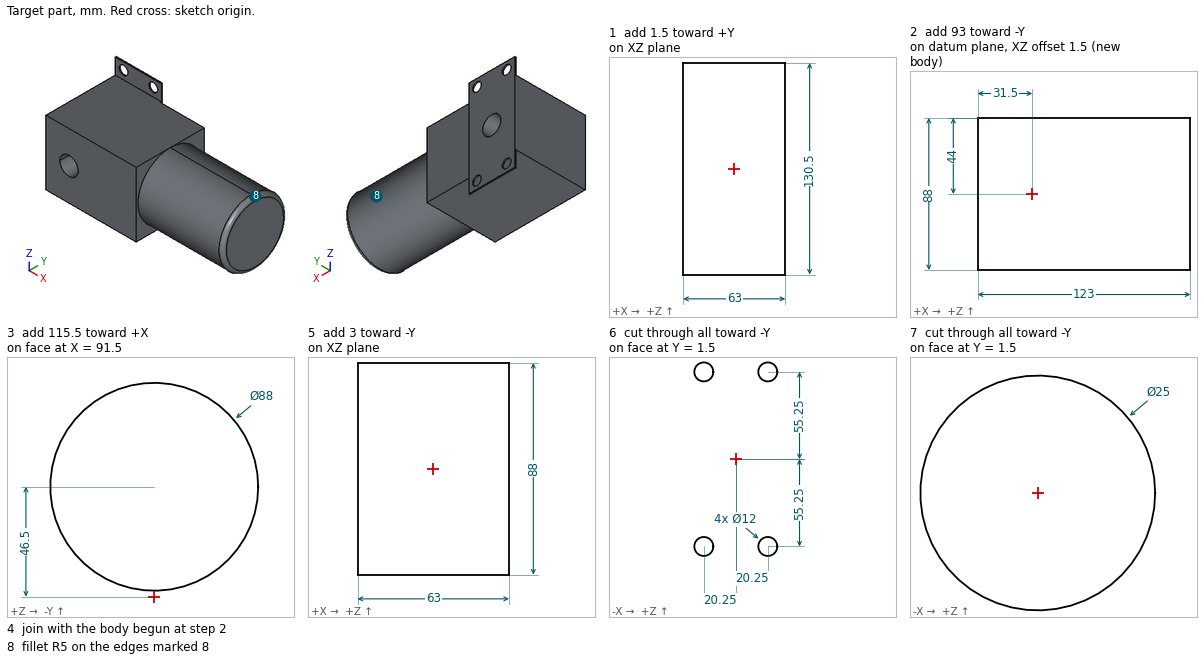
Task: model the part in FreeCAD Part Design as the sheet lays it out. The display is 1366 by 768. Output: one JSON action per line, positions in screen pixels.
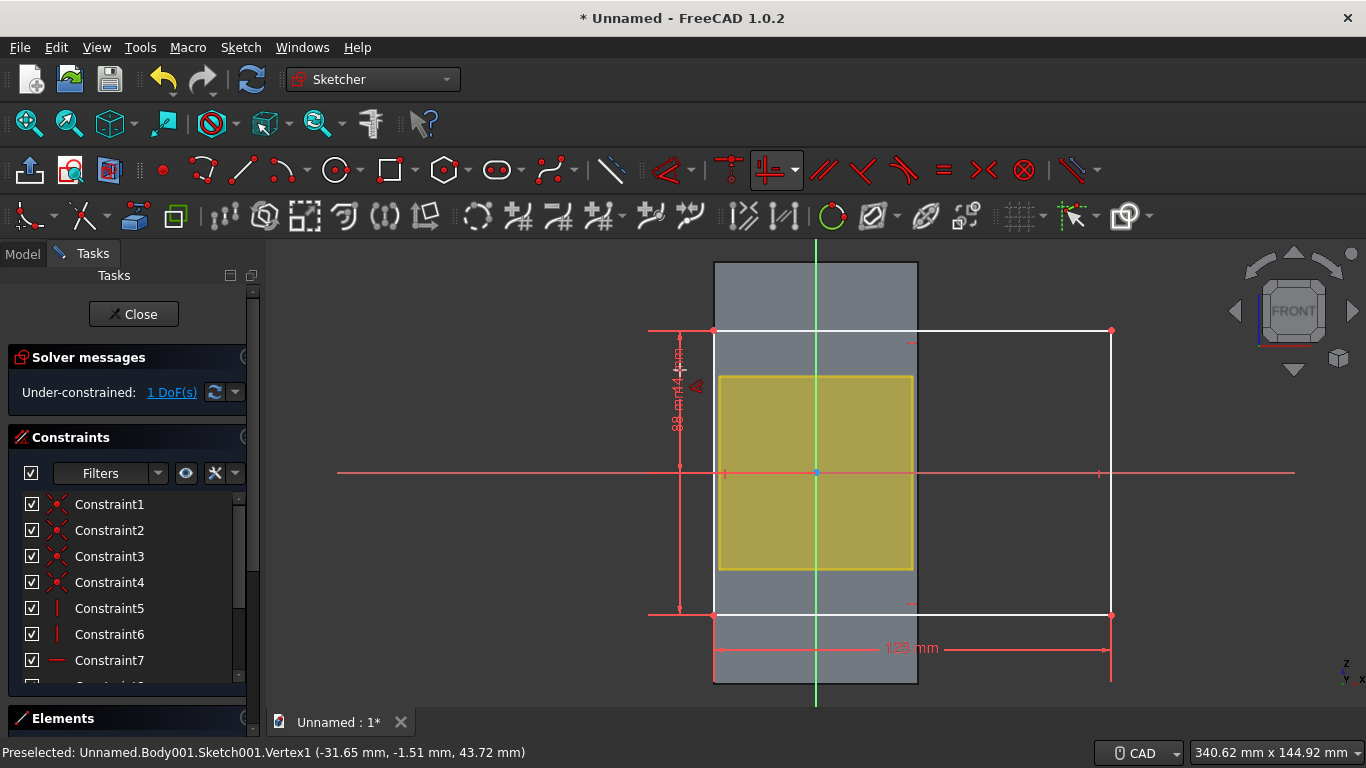
{"action": "left_click", "coordinate": [714, 331]}
{"action": "left_click", "coordinate": [765, 297]}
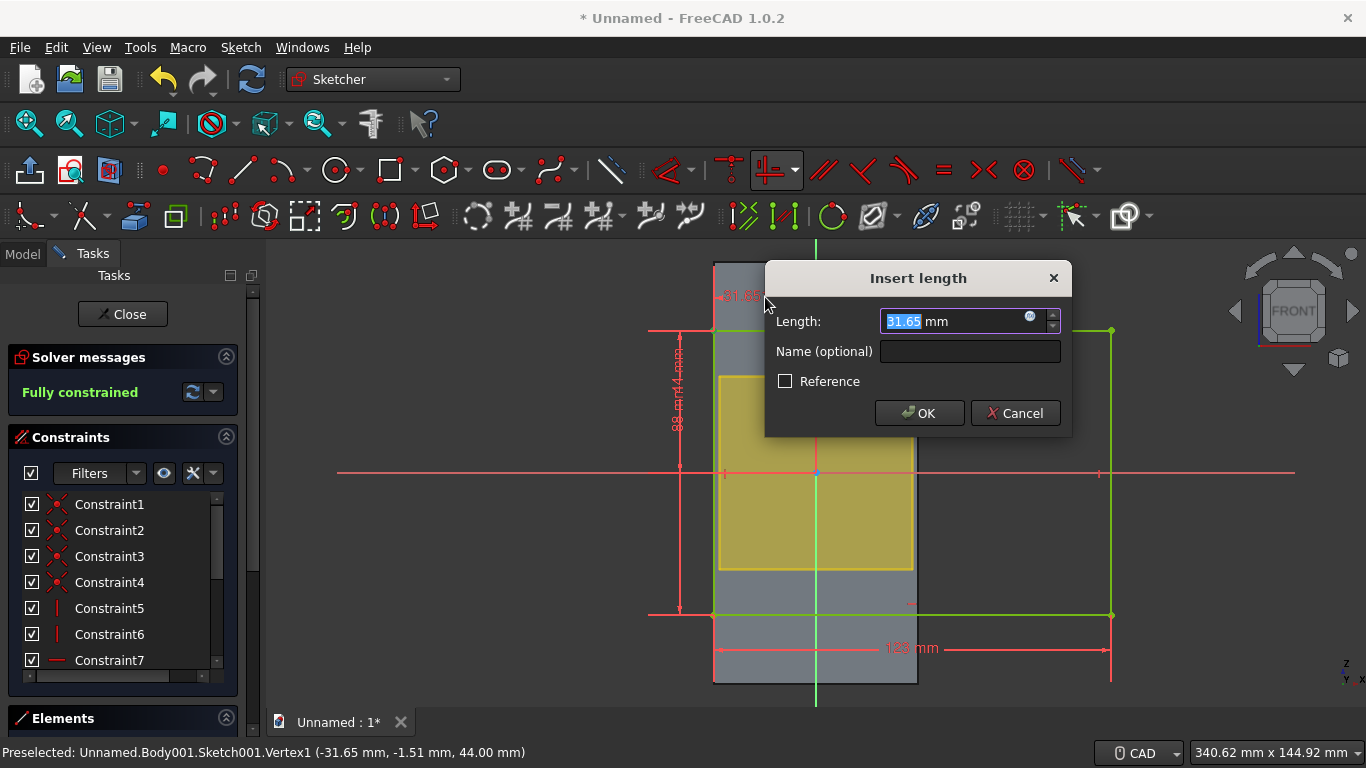
{"action": "type", "text": "31.5"}
{"action": "key", "text": "Return"}
{"action": "key", "text": "Escape"}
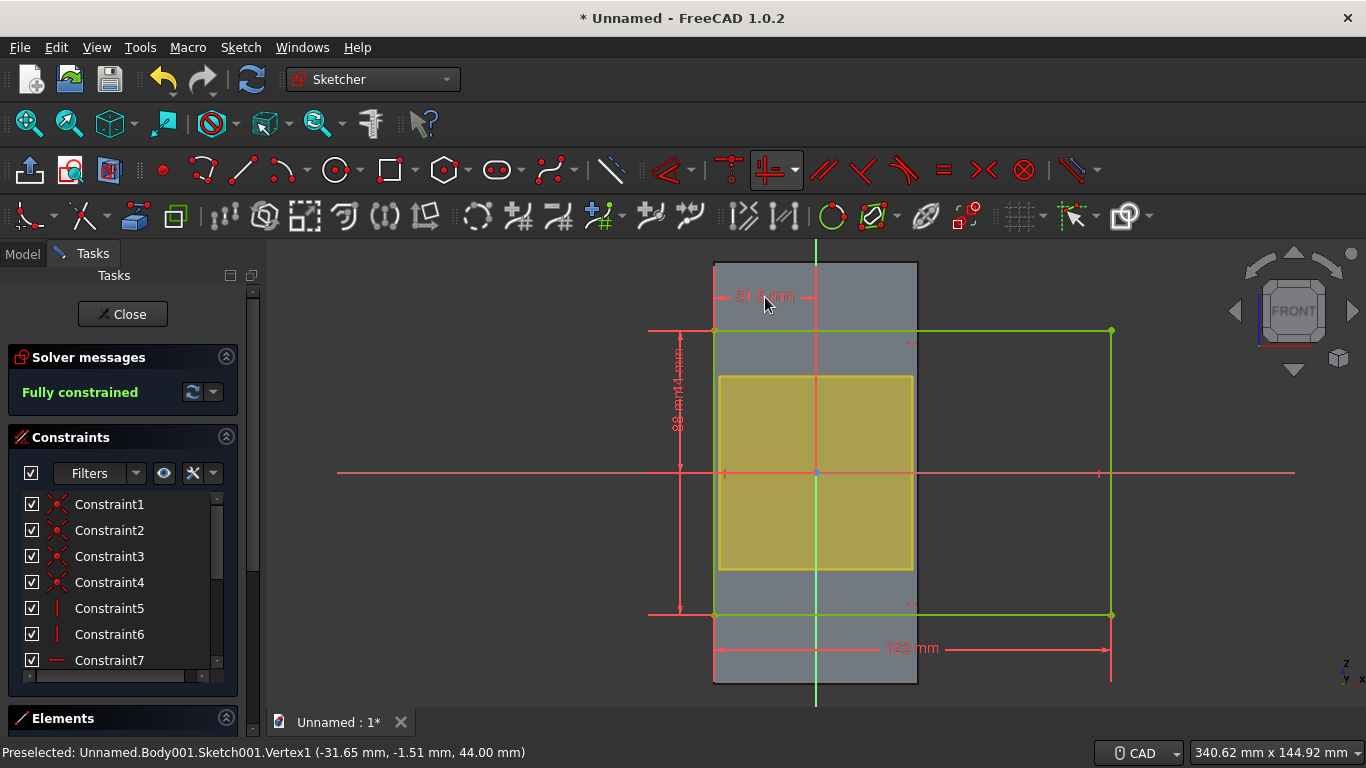
{"action": "left_click", "coordinate": [123, 314]}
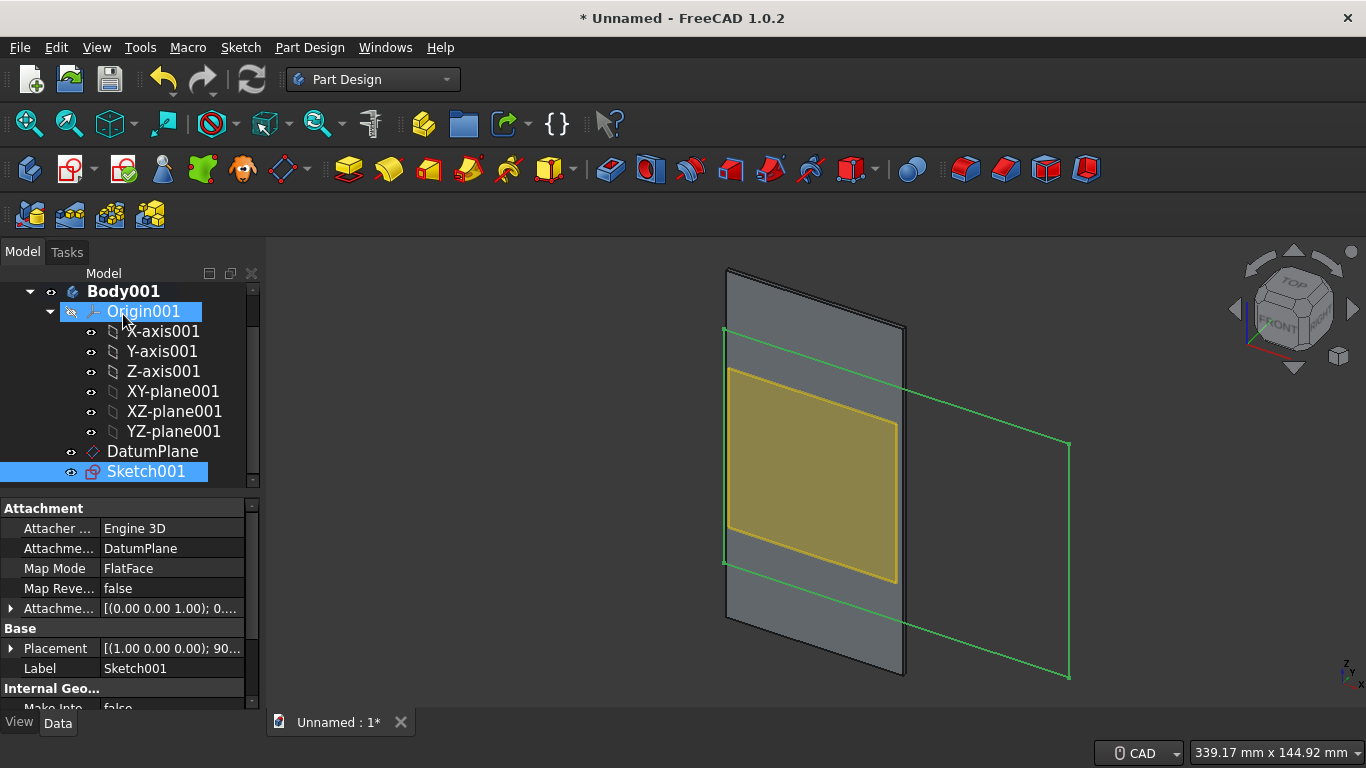
{"action": "left_click", "coordinate": [350, 170]}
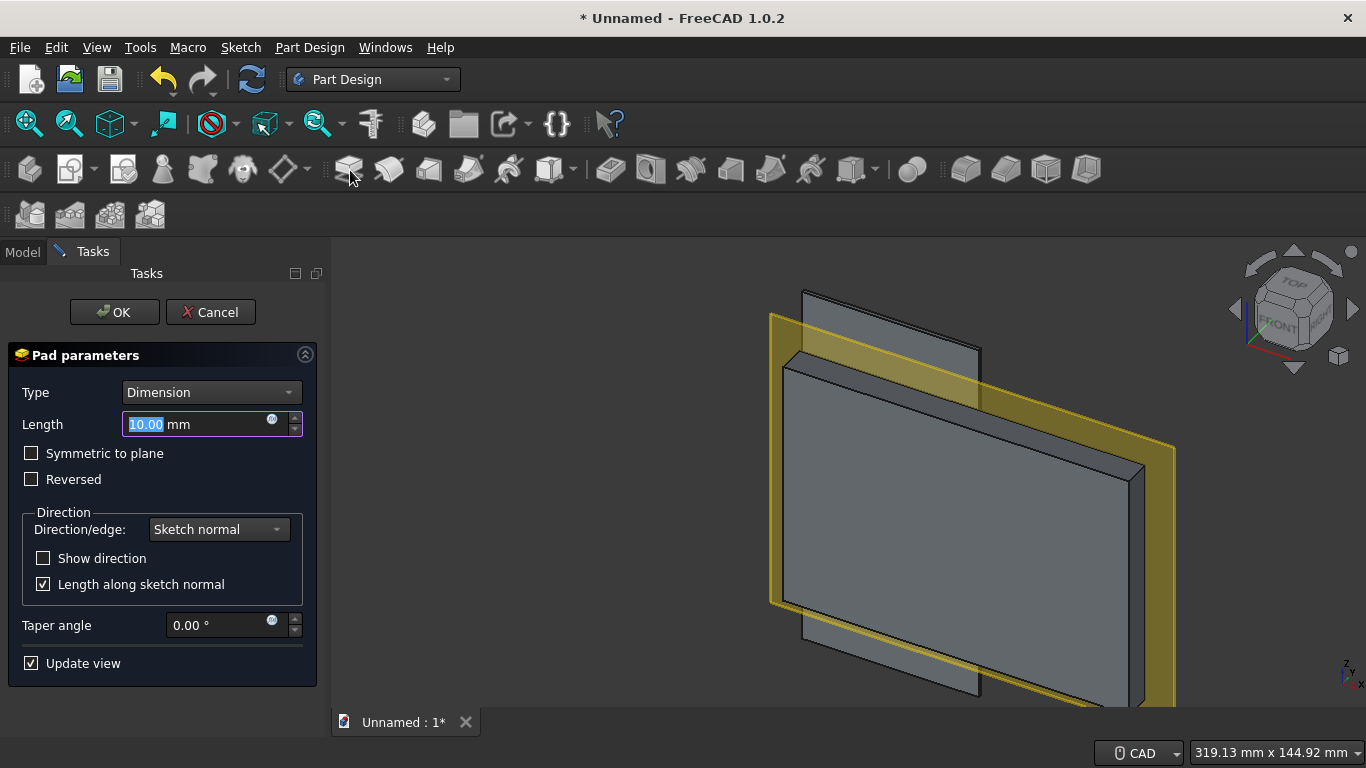
{"action": "type", "text": "93"}
{"action": "key", "text": "Tab"}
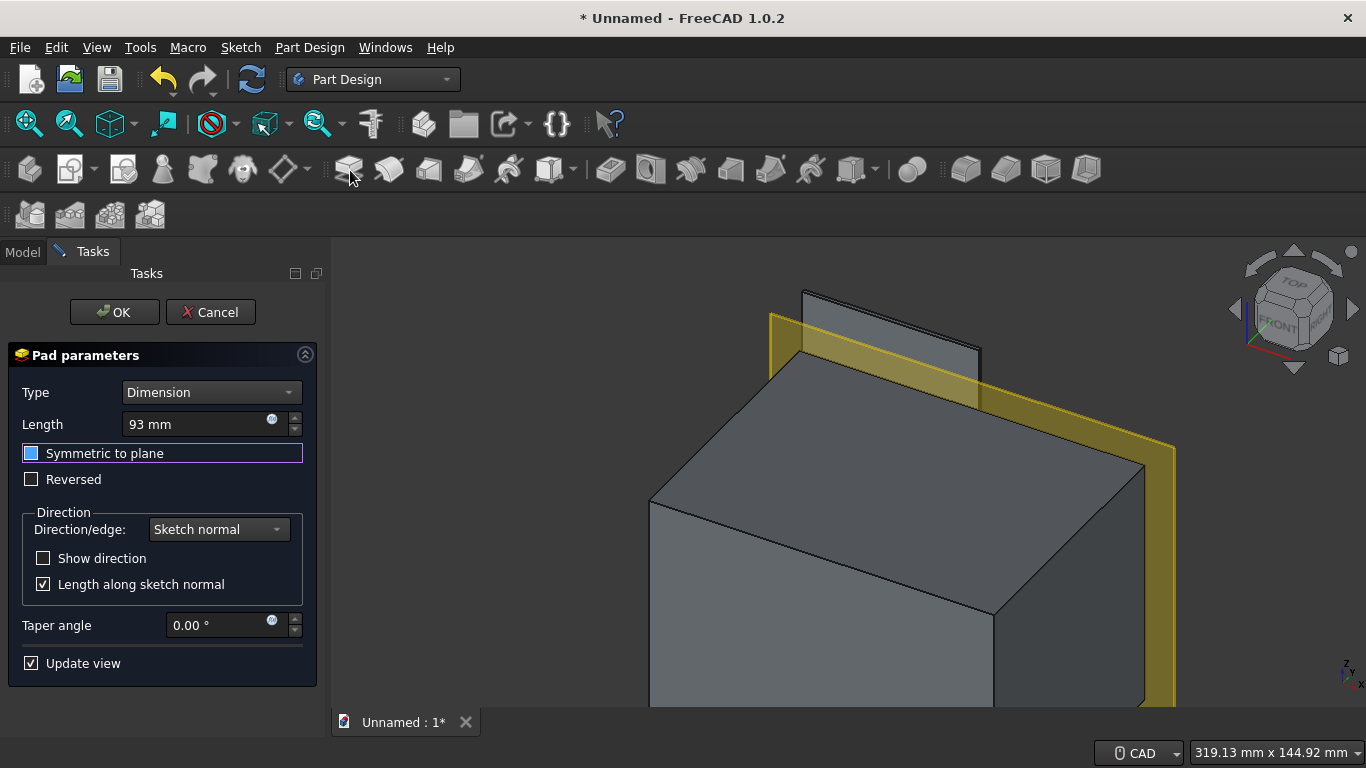
{"action": "left_click", "coordinate": [115, 312]}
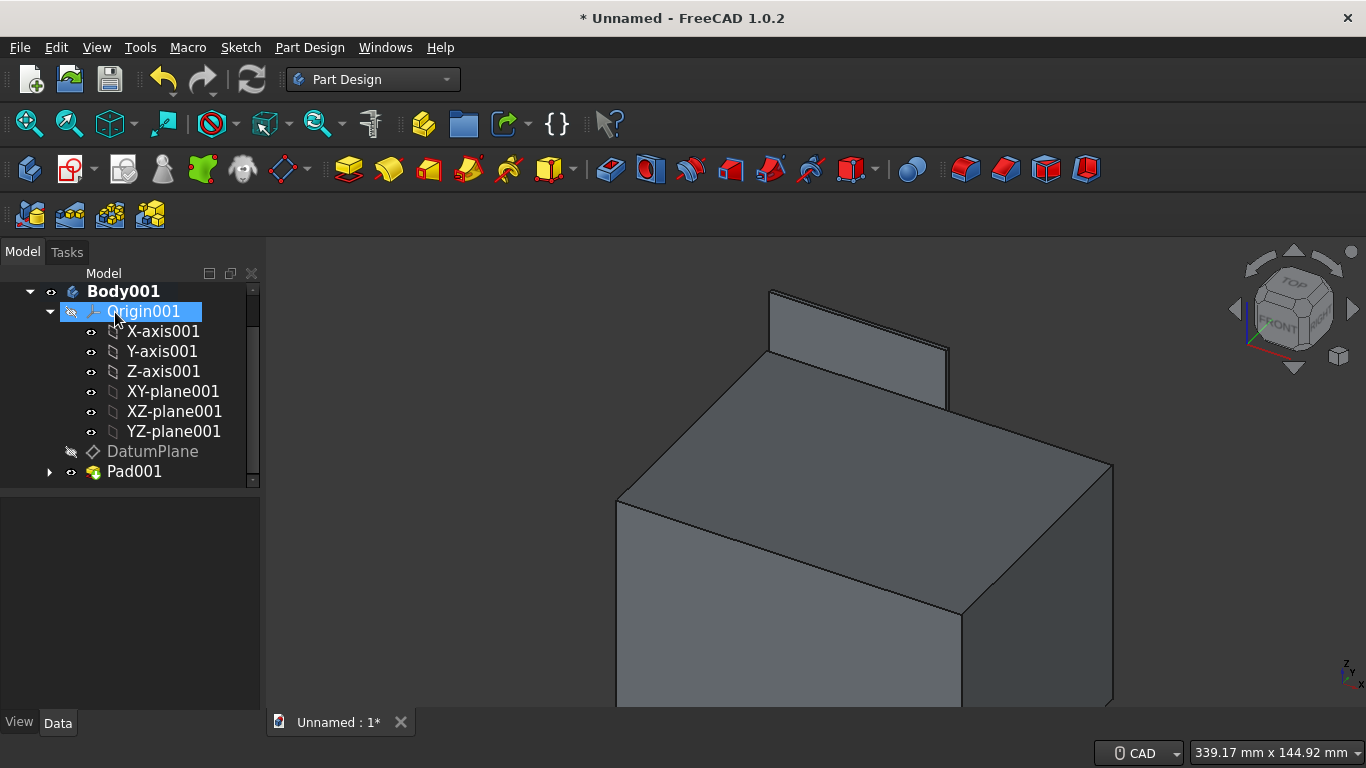
{"action": "left_click", "coordinate": [30, 124]}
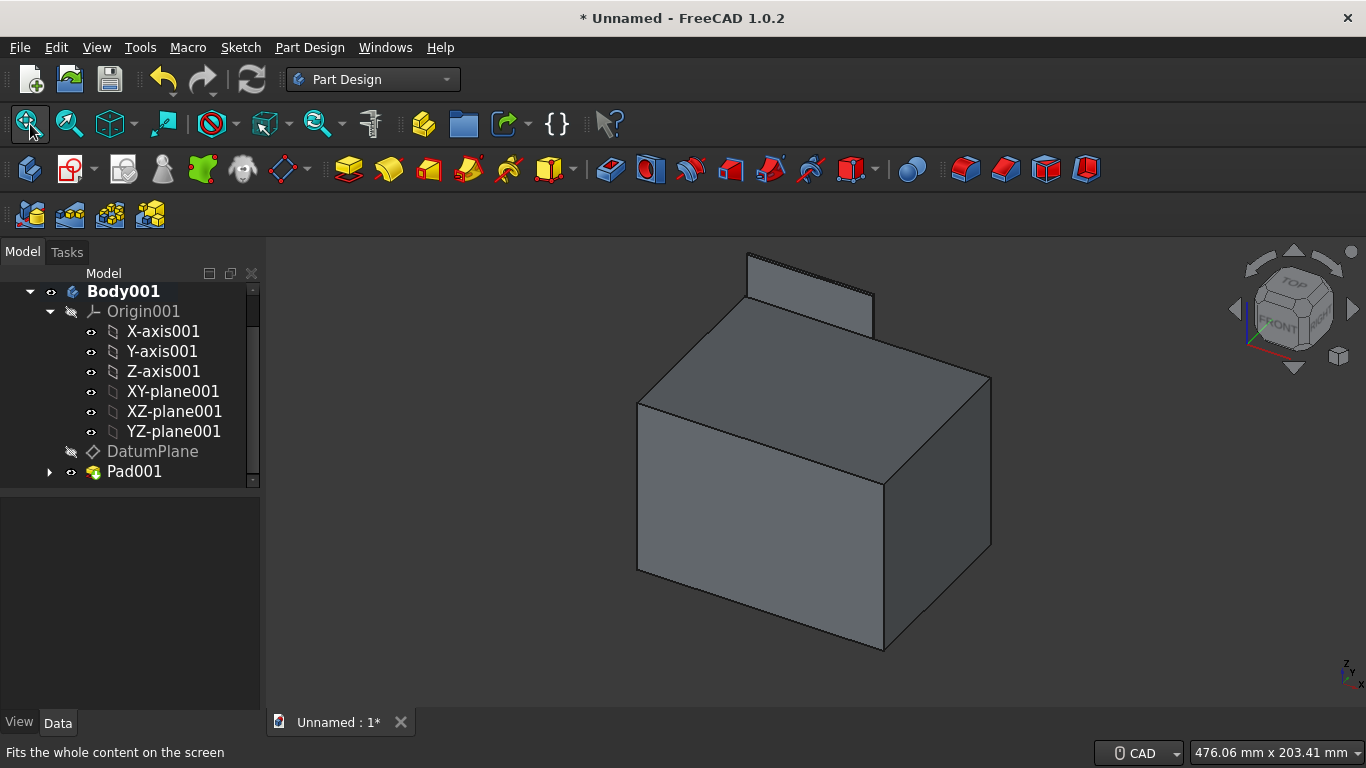
{"action": "left_click", "coordinate": [937, 513]}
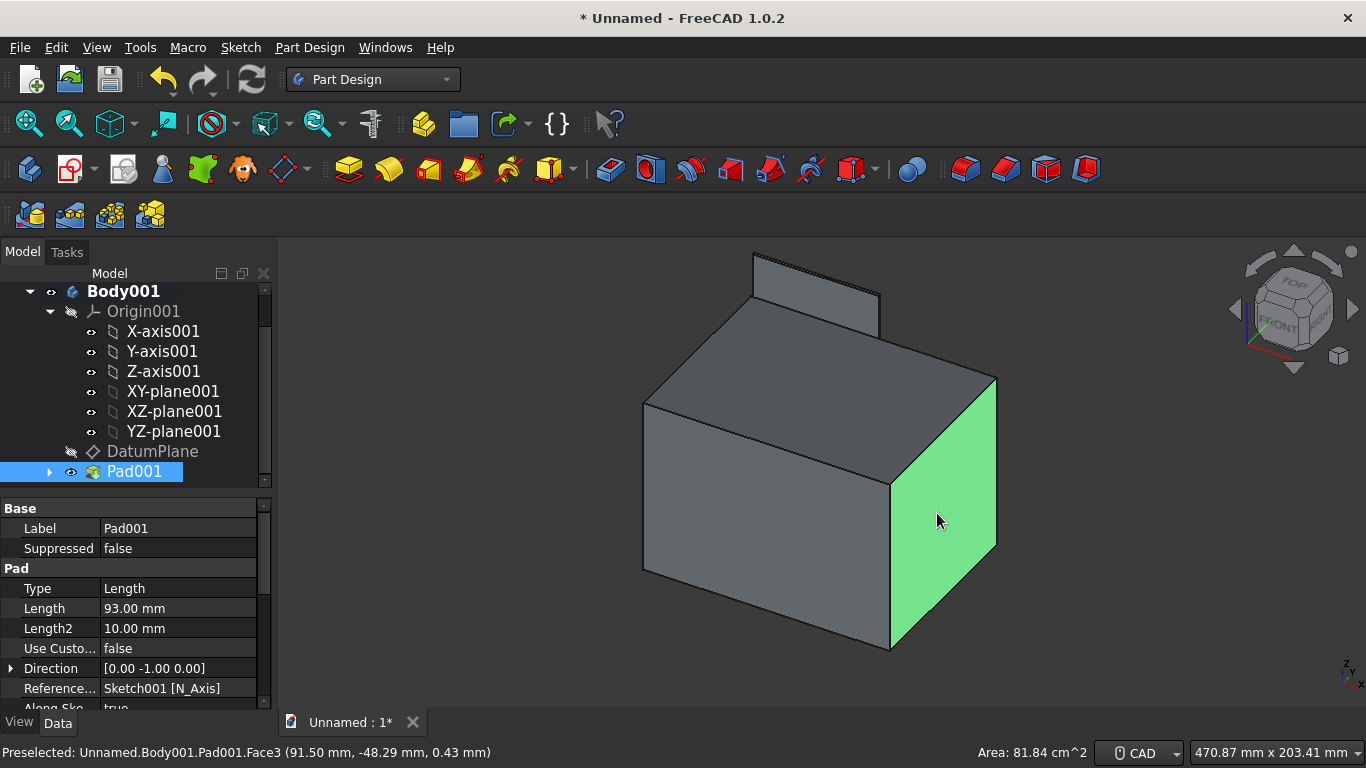
{"action": "left_click", "coordinate": [70, 170]}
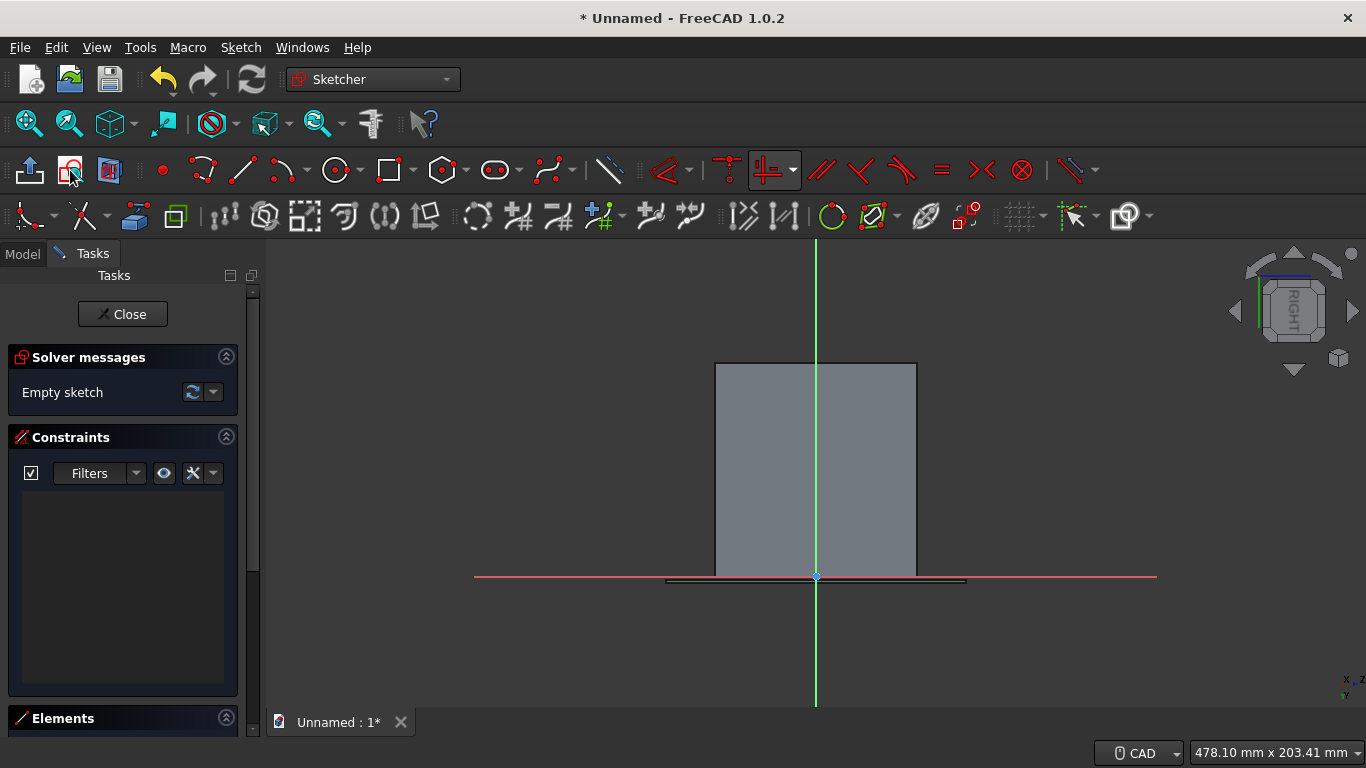
{"action": "scroll", "coordinate": [955, 471], "scroll_direction": "up", "scroll_amount": 2}